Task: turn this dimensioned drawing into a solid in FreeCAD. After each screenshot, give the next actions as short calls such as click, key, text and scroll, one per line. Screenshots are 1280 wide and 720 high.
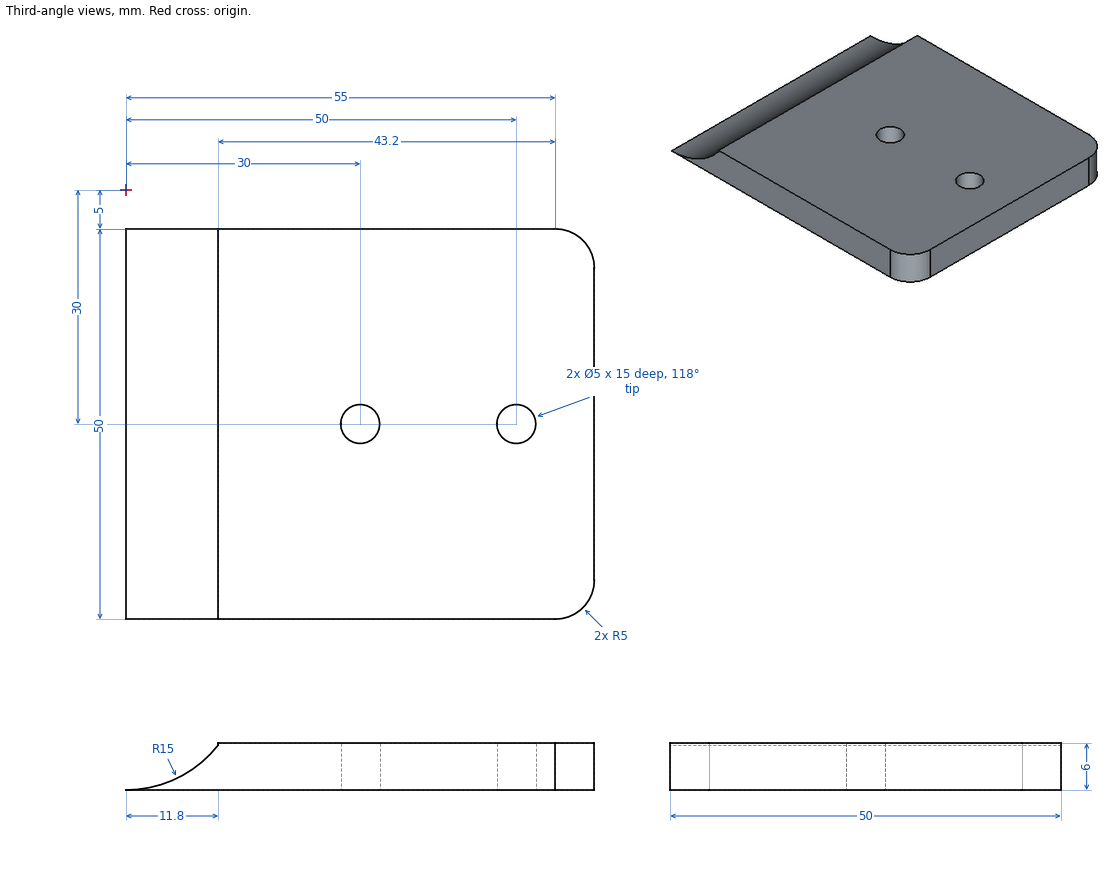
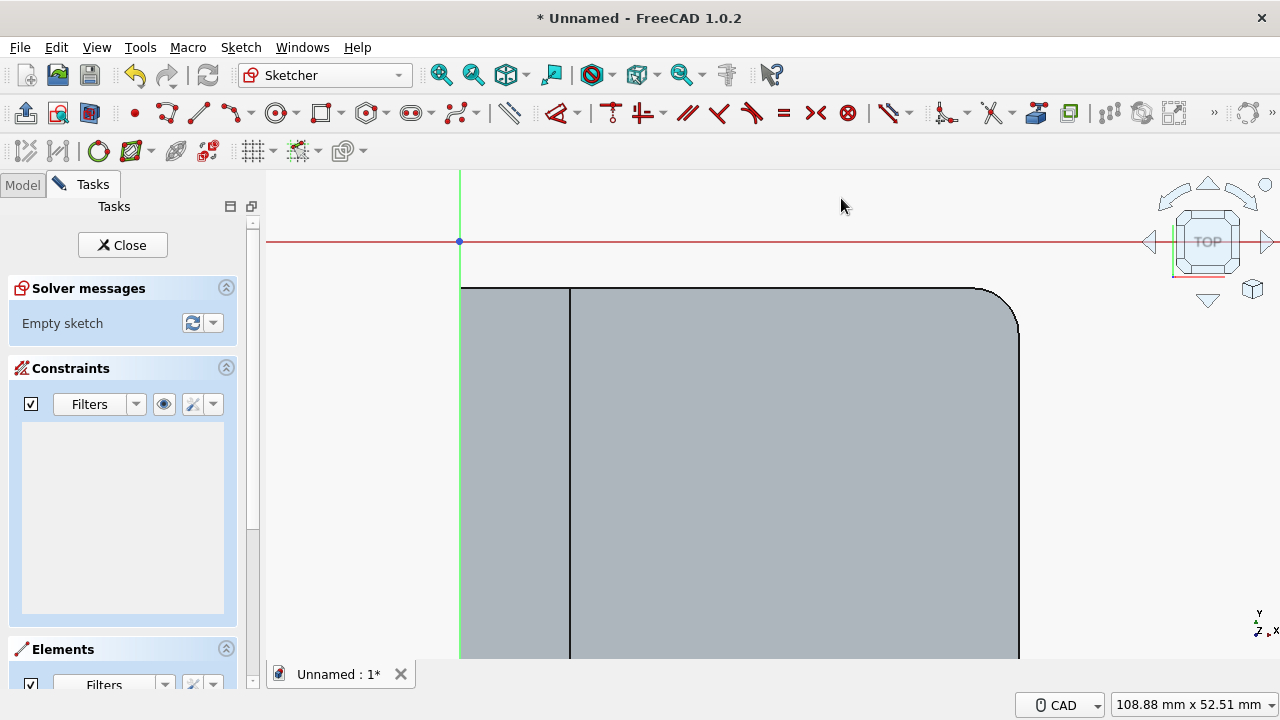
click(276, 114)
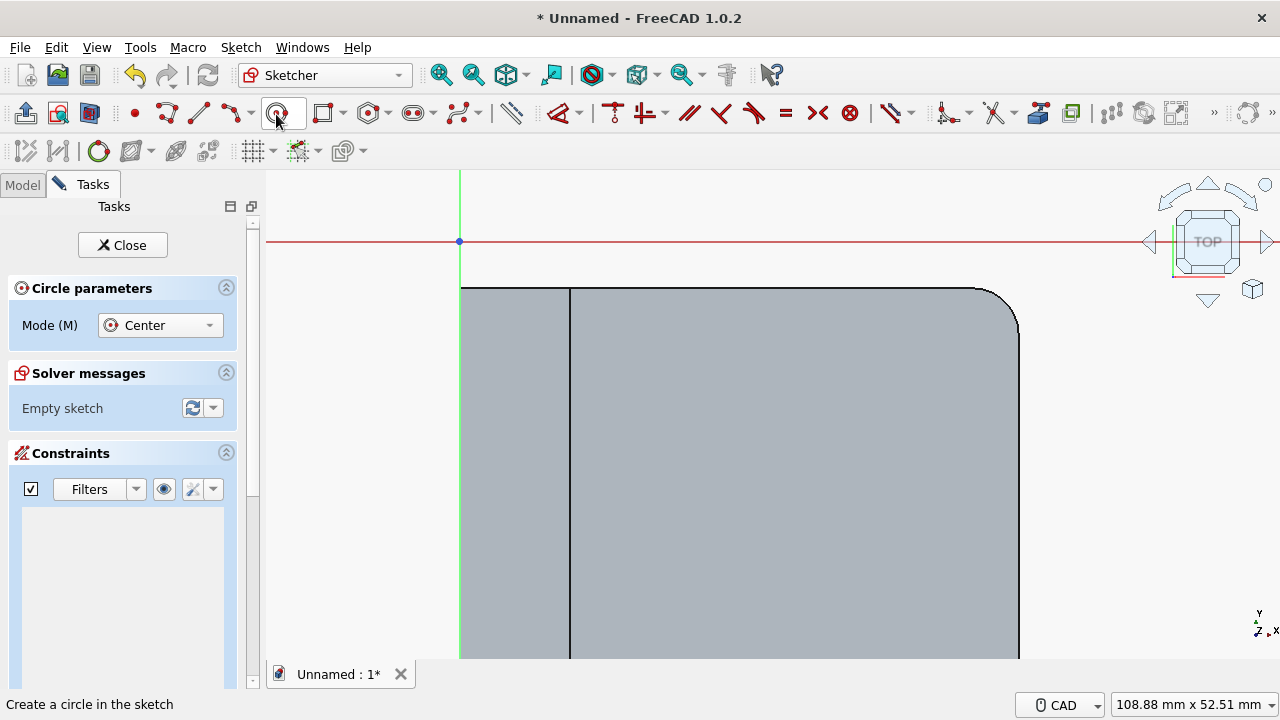
click(926, 521)
move(942, 504)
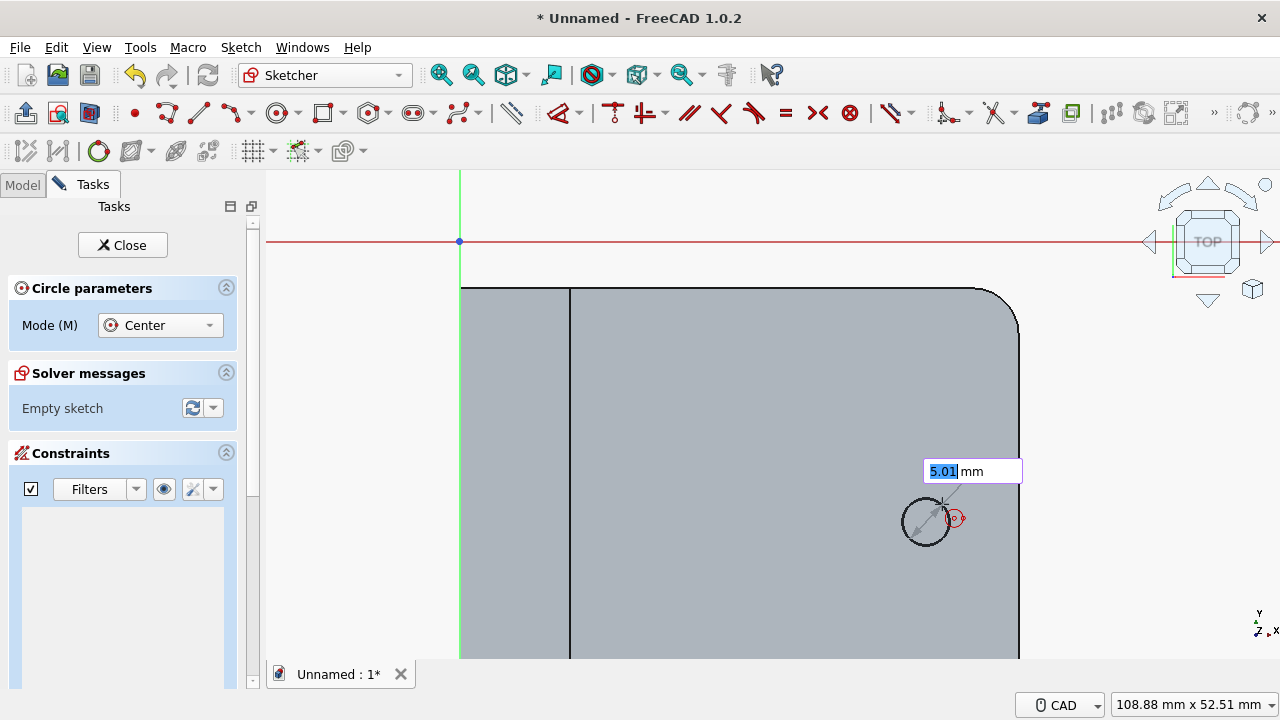
text(5)
key(Return)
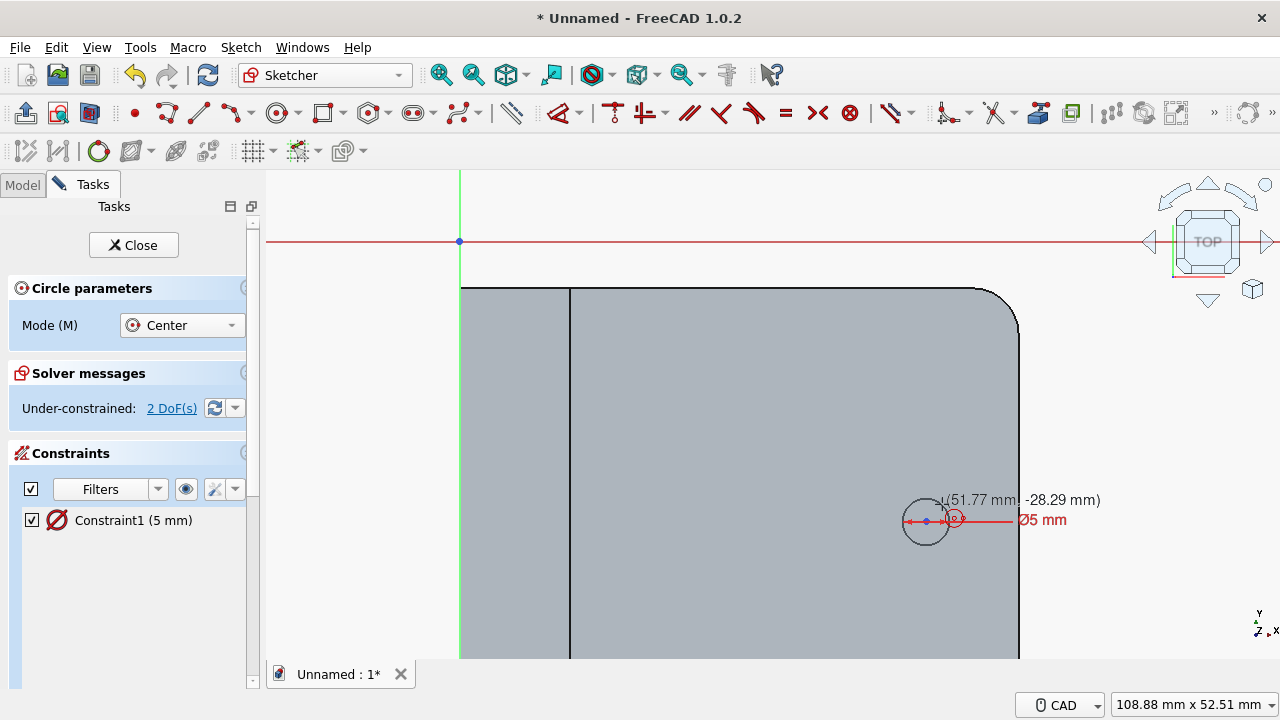
click(739, 521)
move(756, 504)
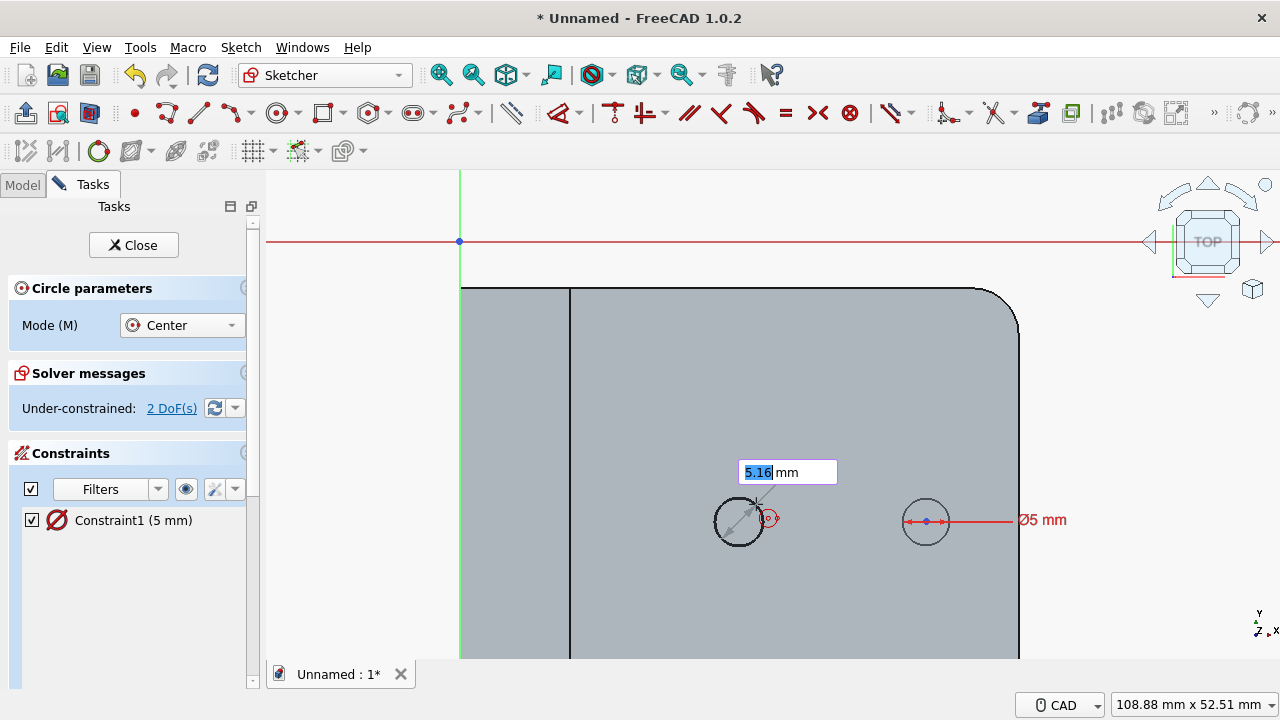
text(5)
key(Return)
key(Escape)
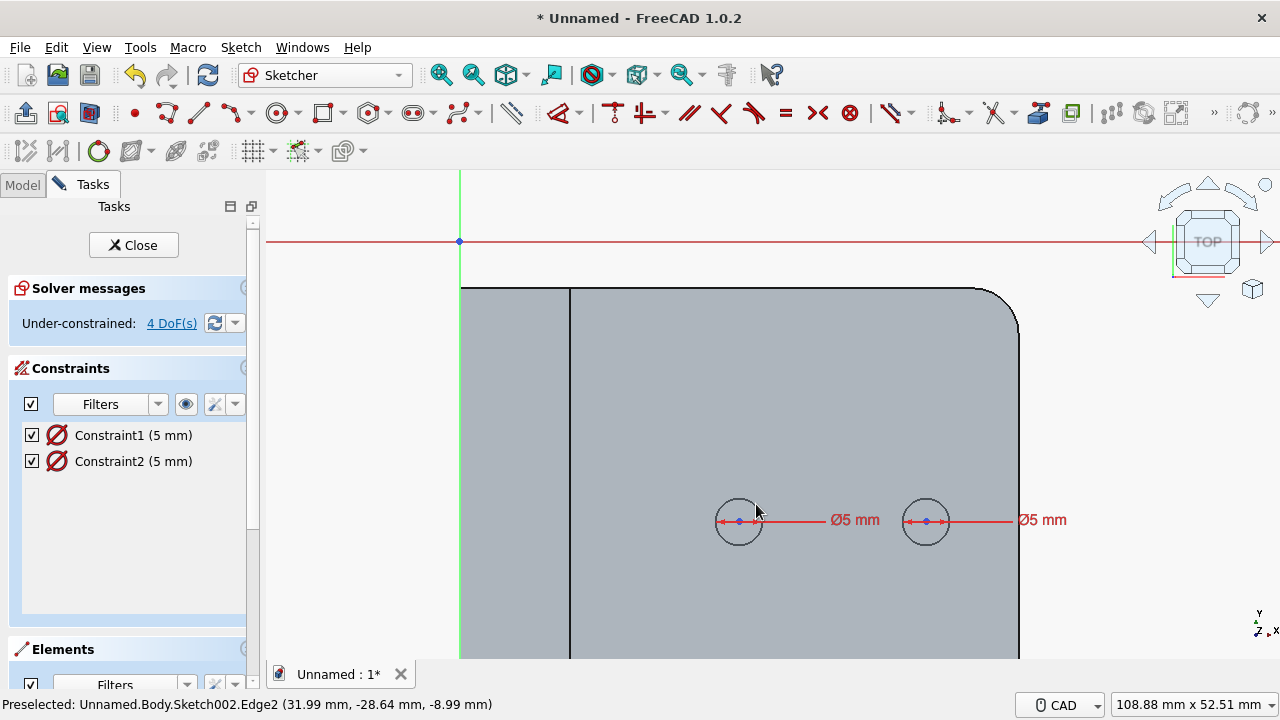
click(926, 522)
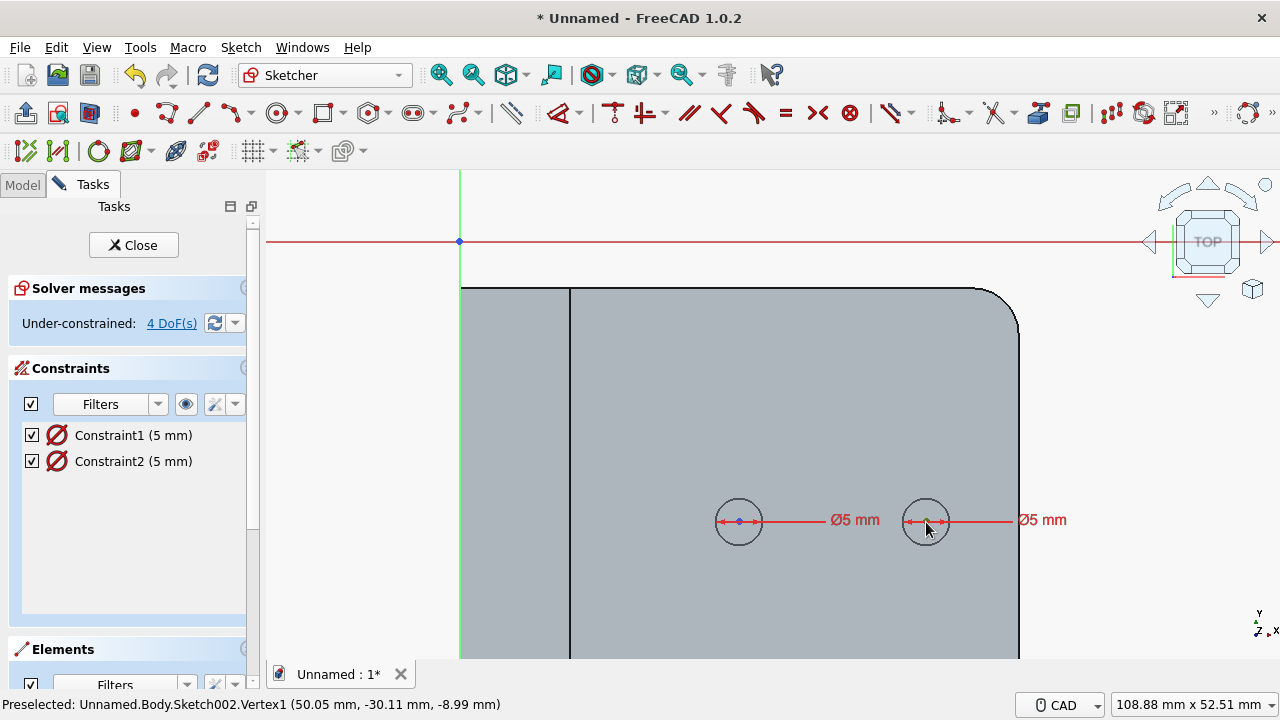
click(739, 522)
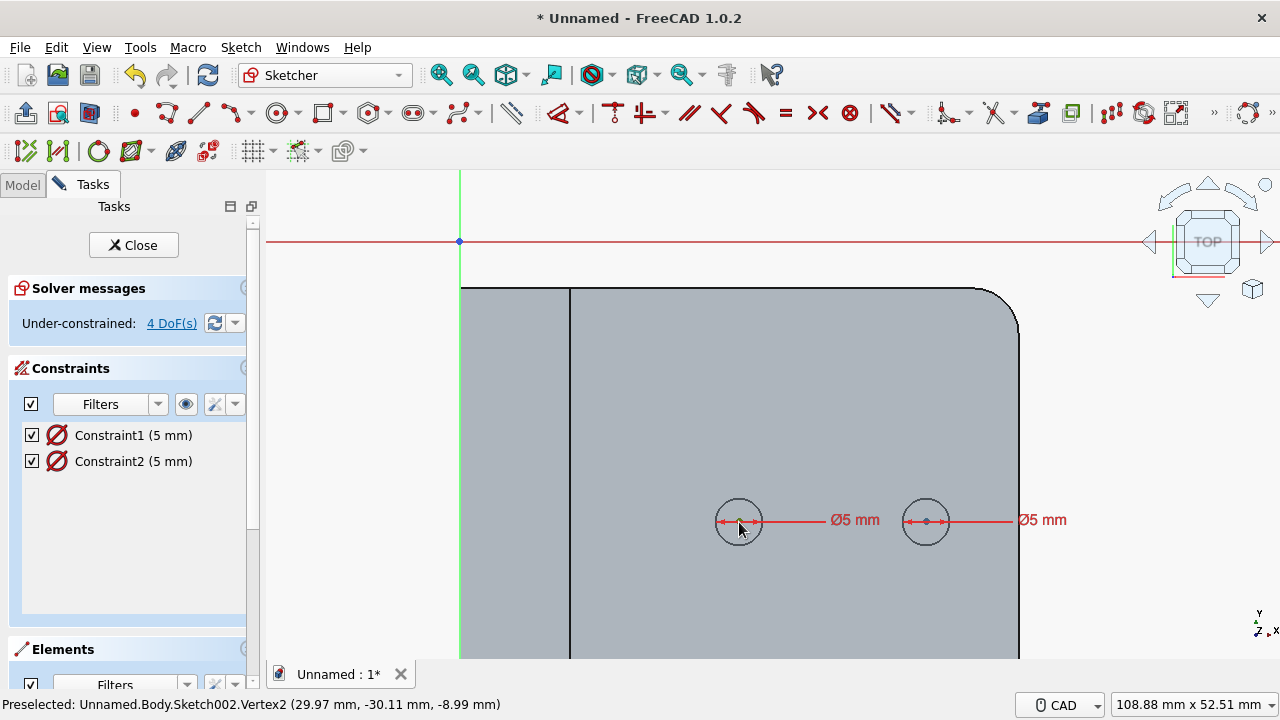
click(668, 114)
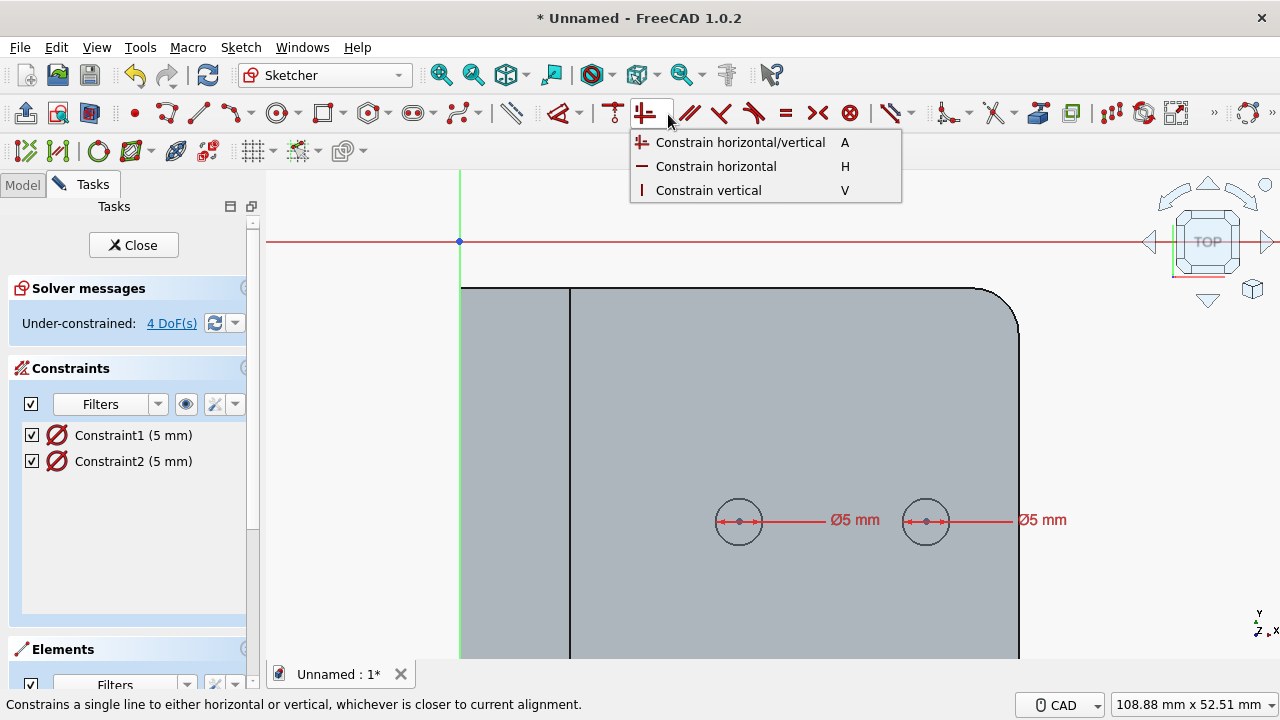
click(766, 166)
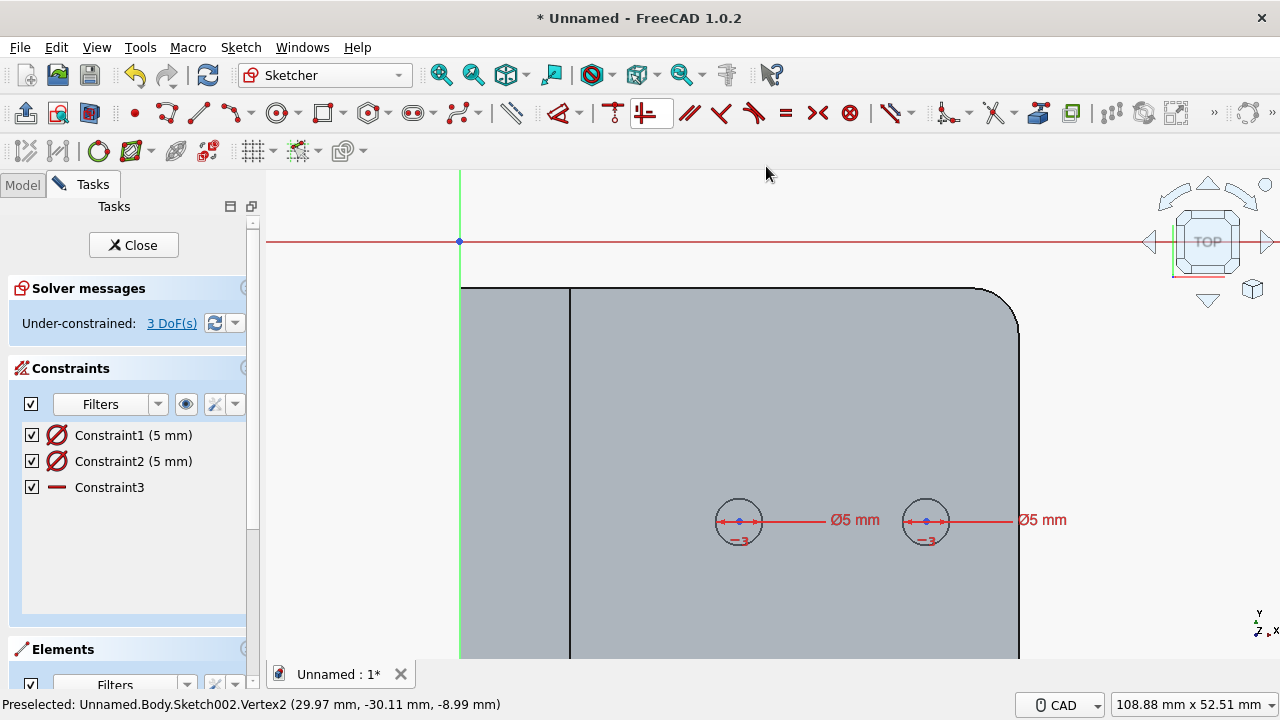
click(558, 114)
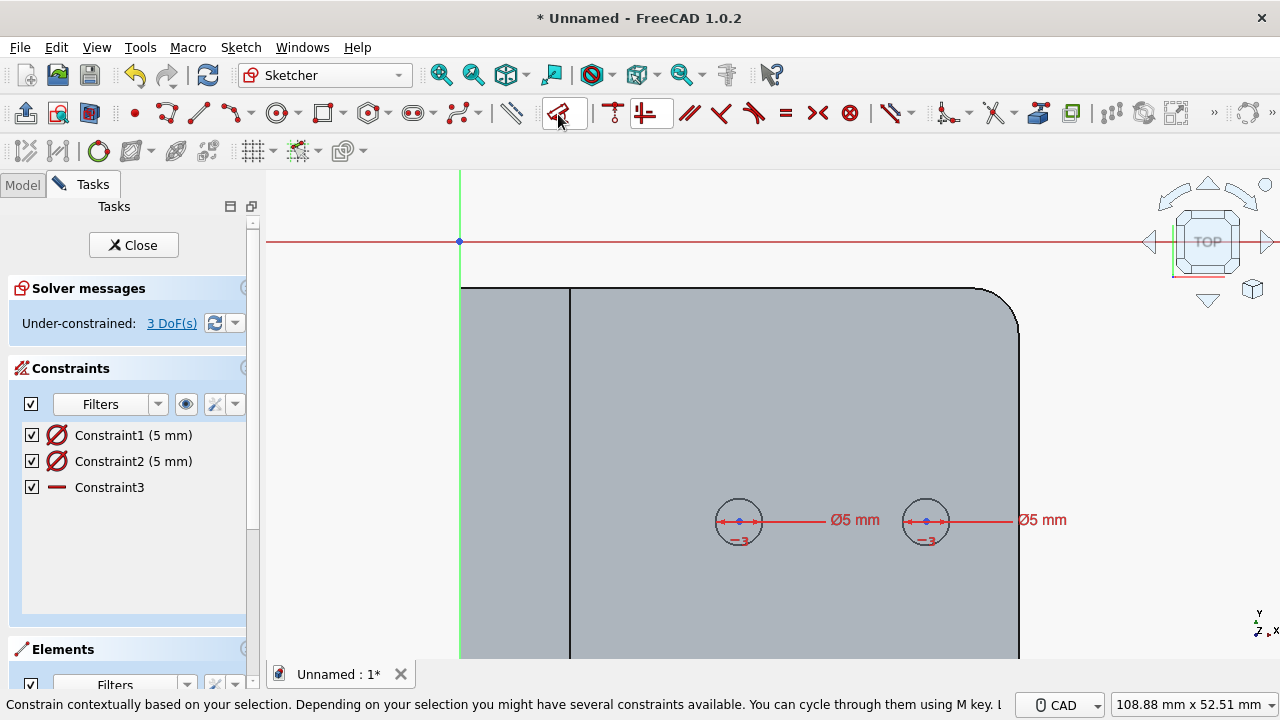
click(926, 522)
click(693, 208)